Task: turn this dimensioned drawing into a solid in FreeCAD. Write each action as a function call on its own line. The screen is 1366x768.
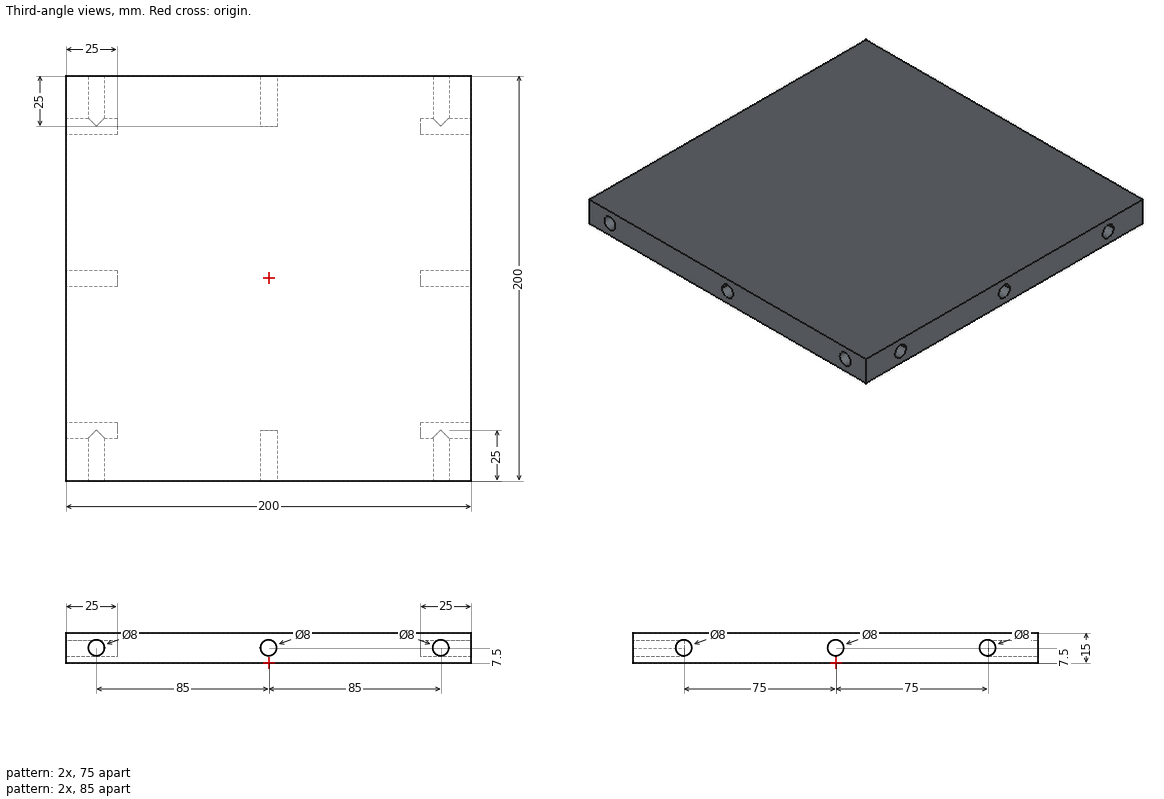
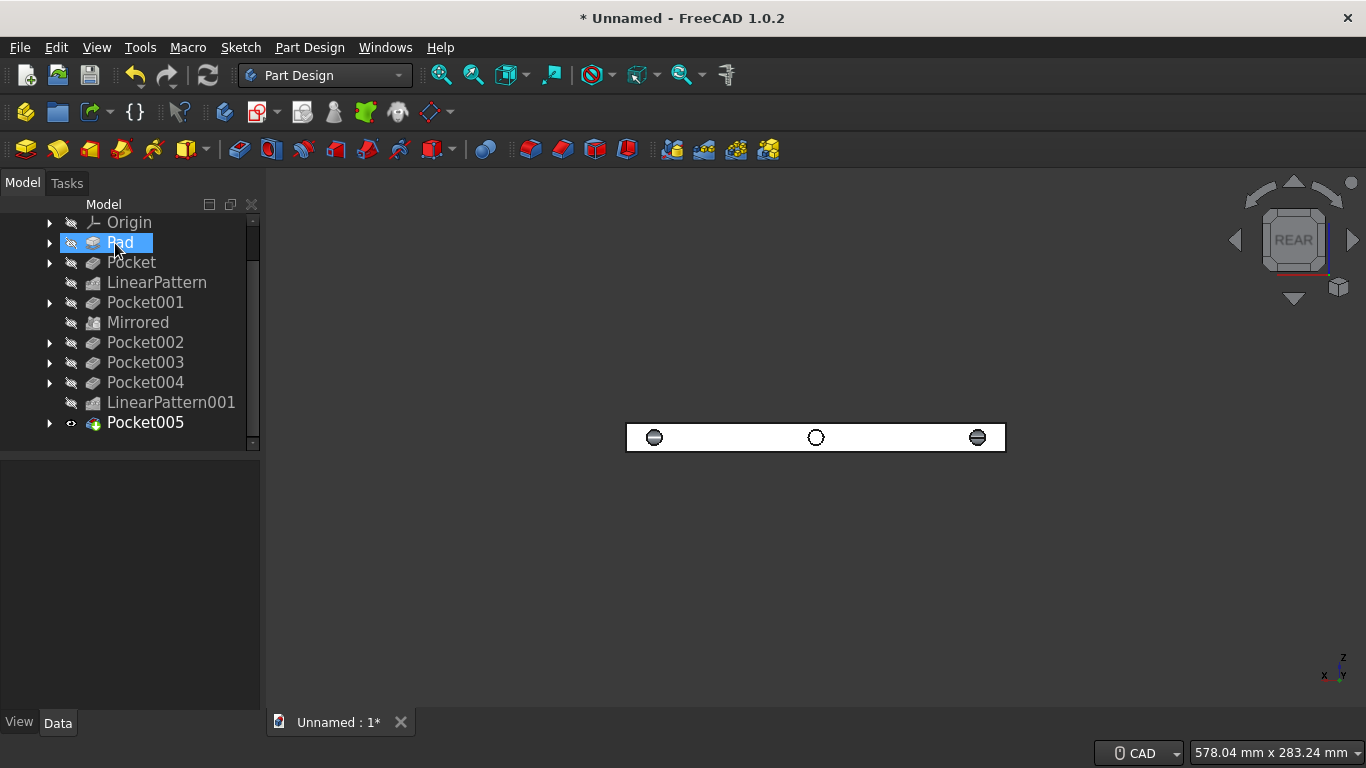
key(v)
key(f)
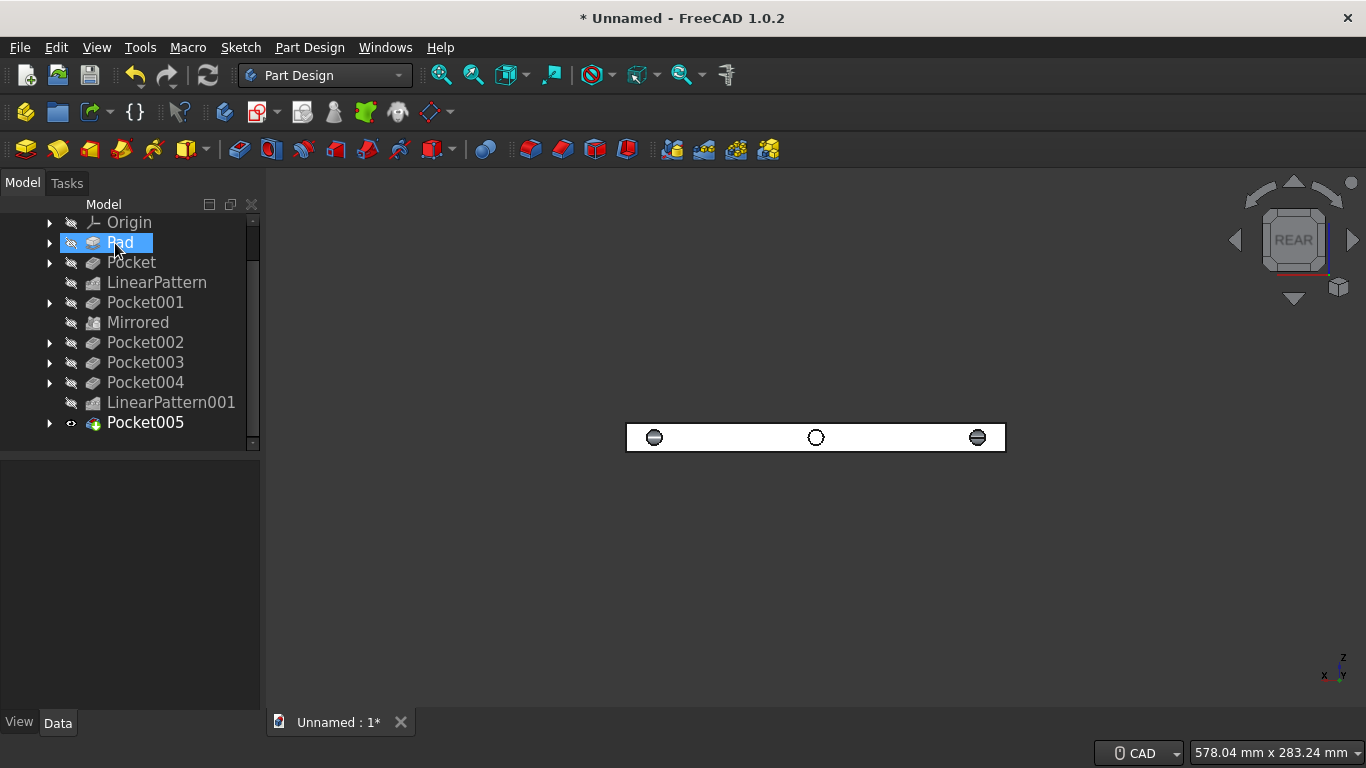
click(116, 383)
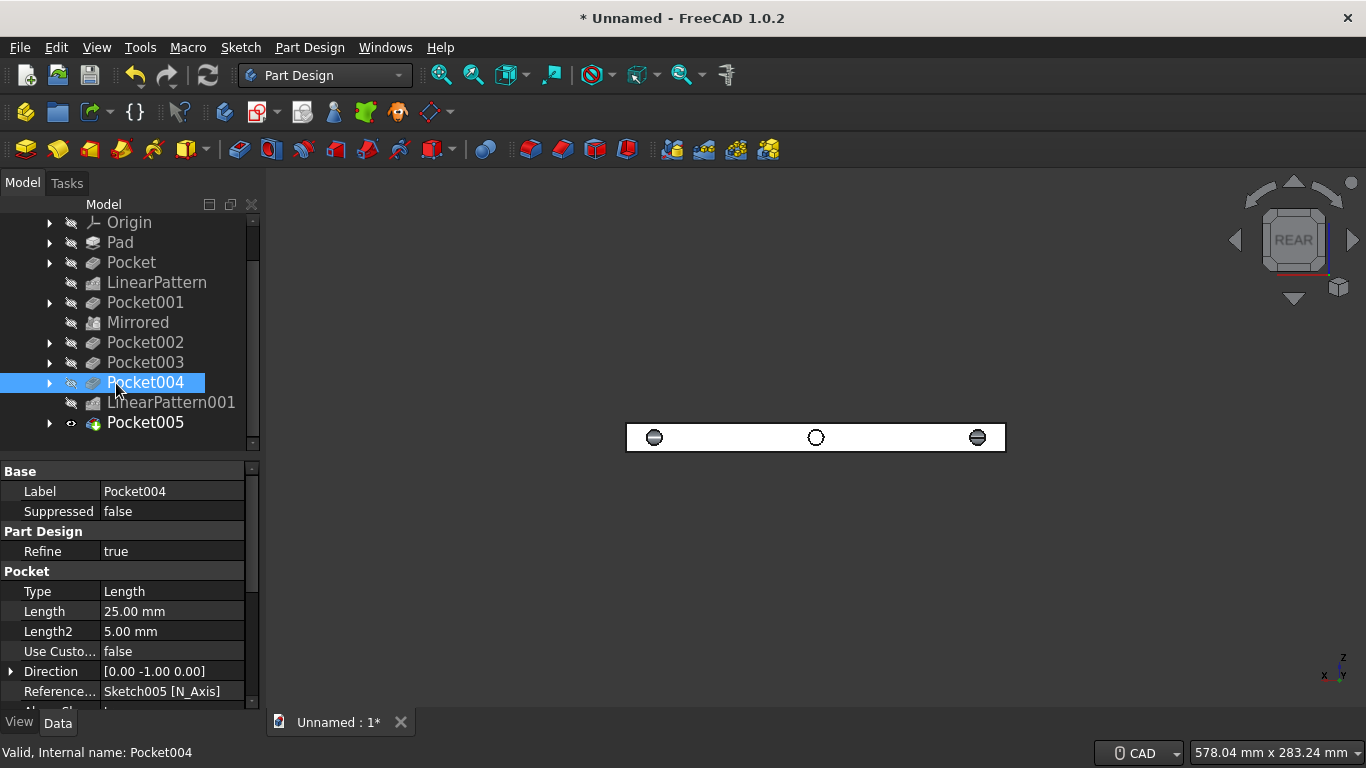
click(672, 150)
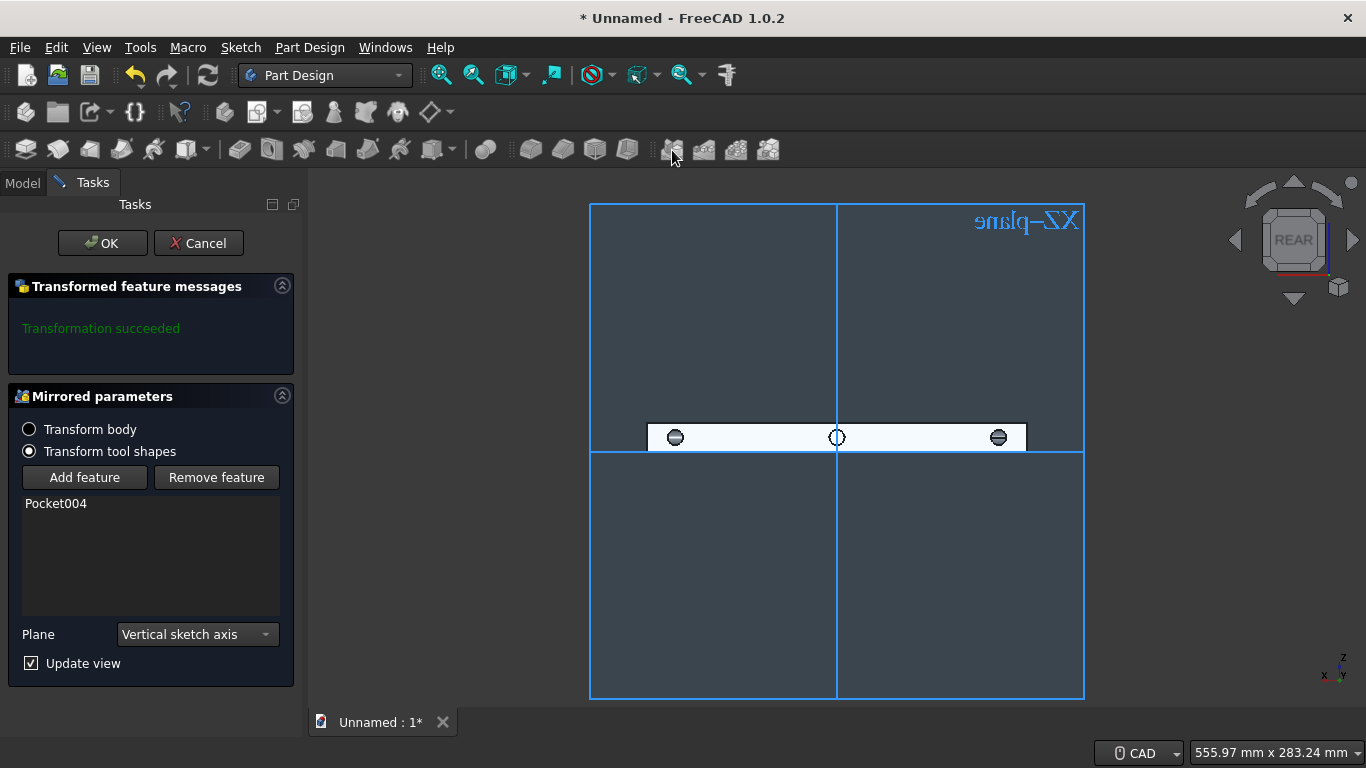
click(198, 634)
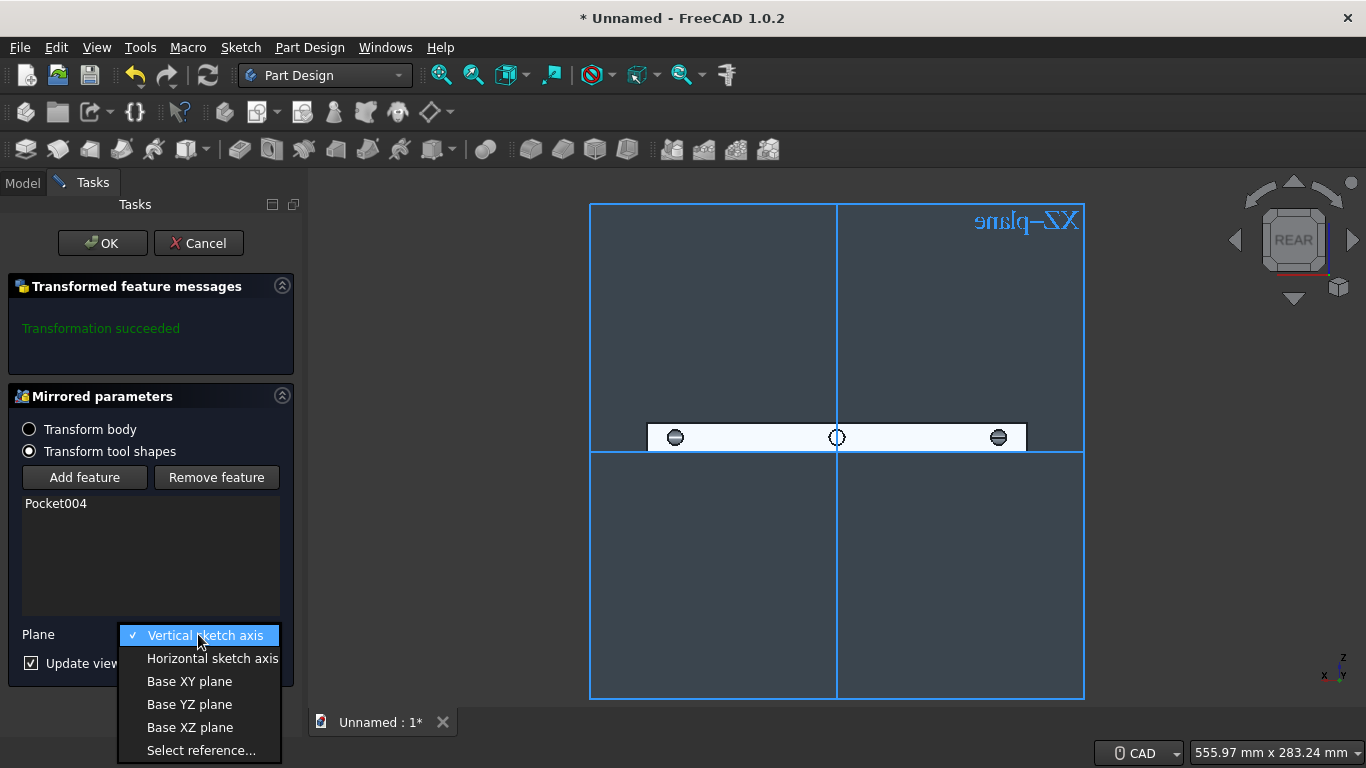
click(198, 728)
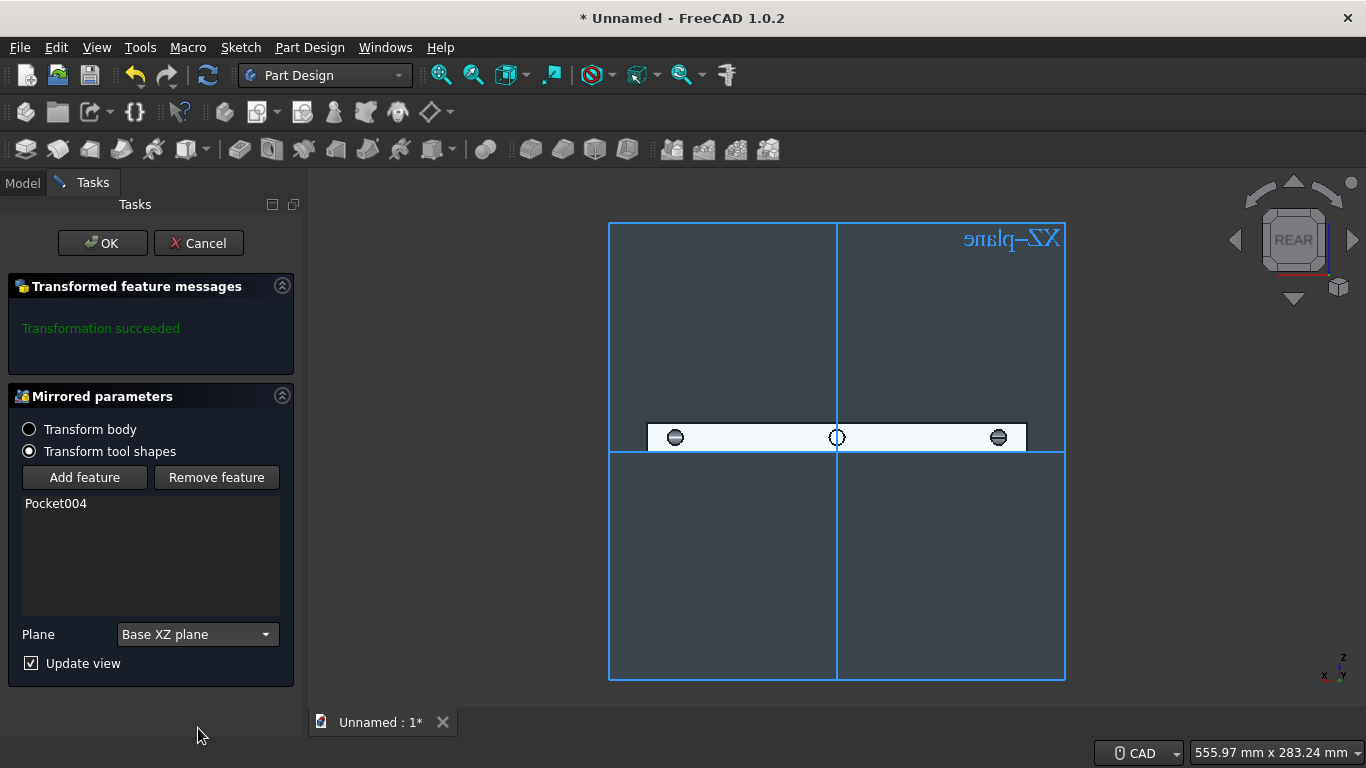
click(103, 243)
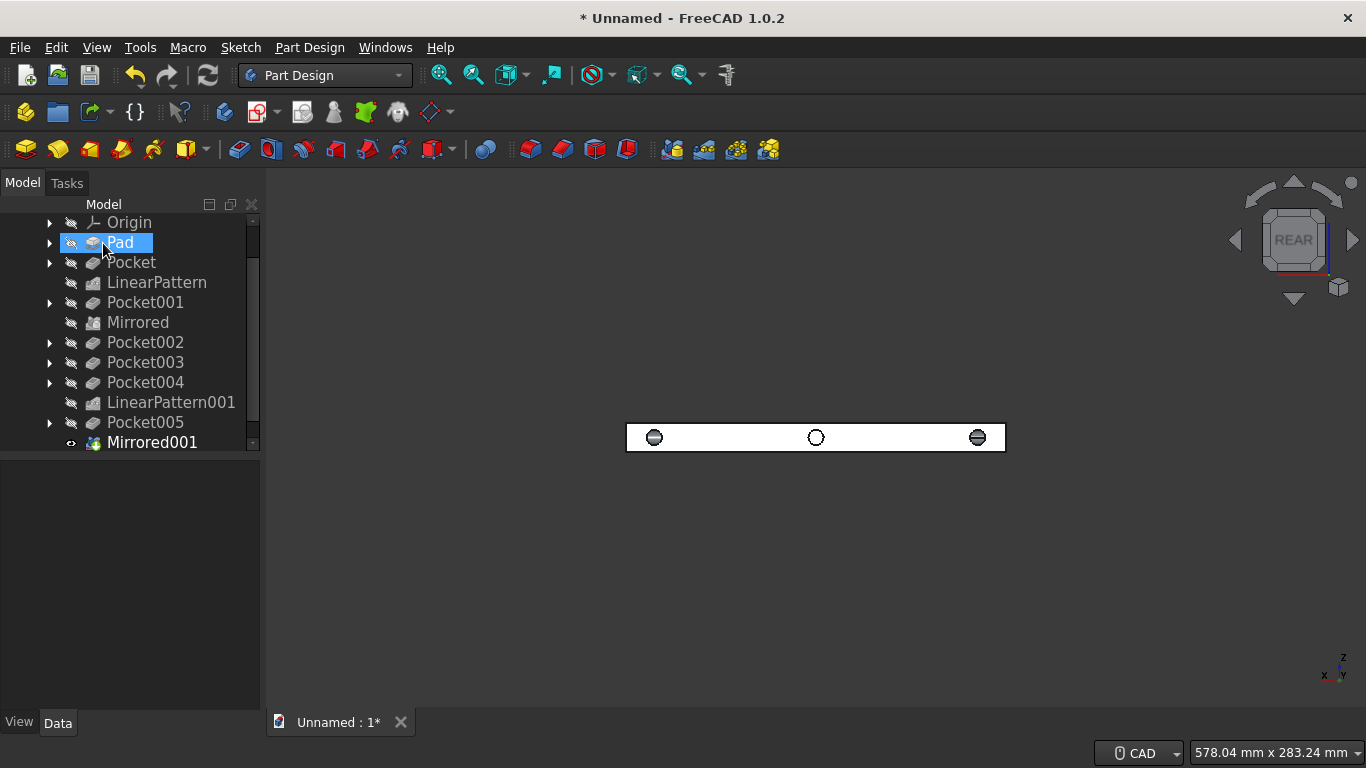
key(v)
key(f)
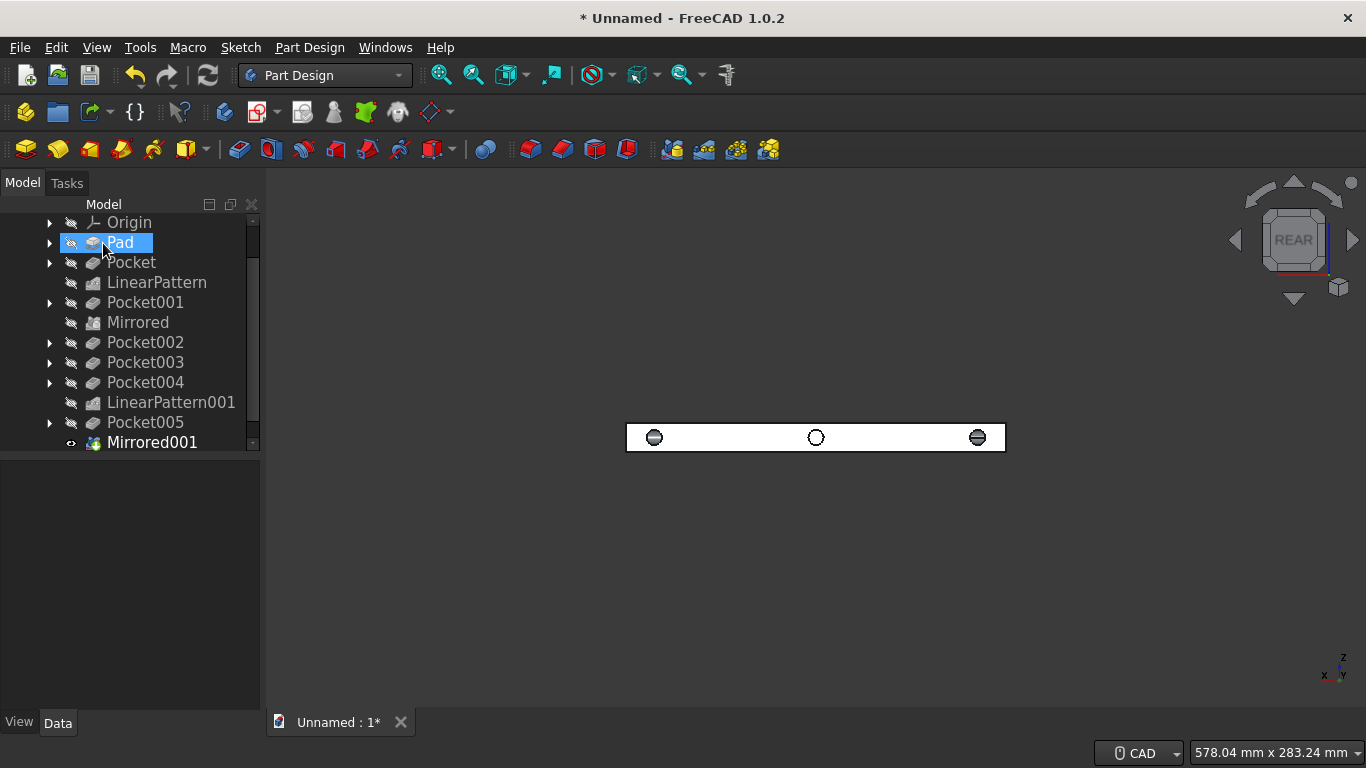
key(0)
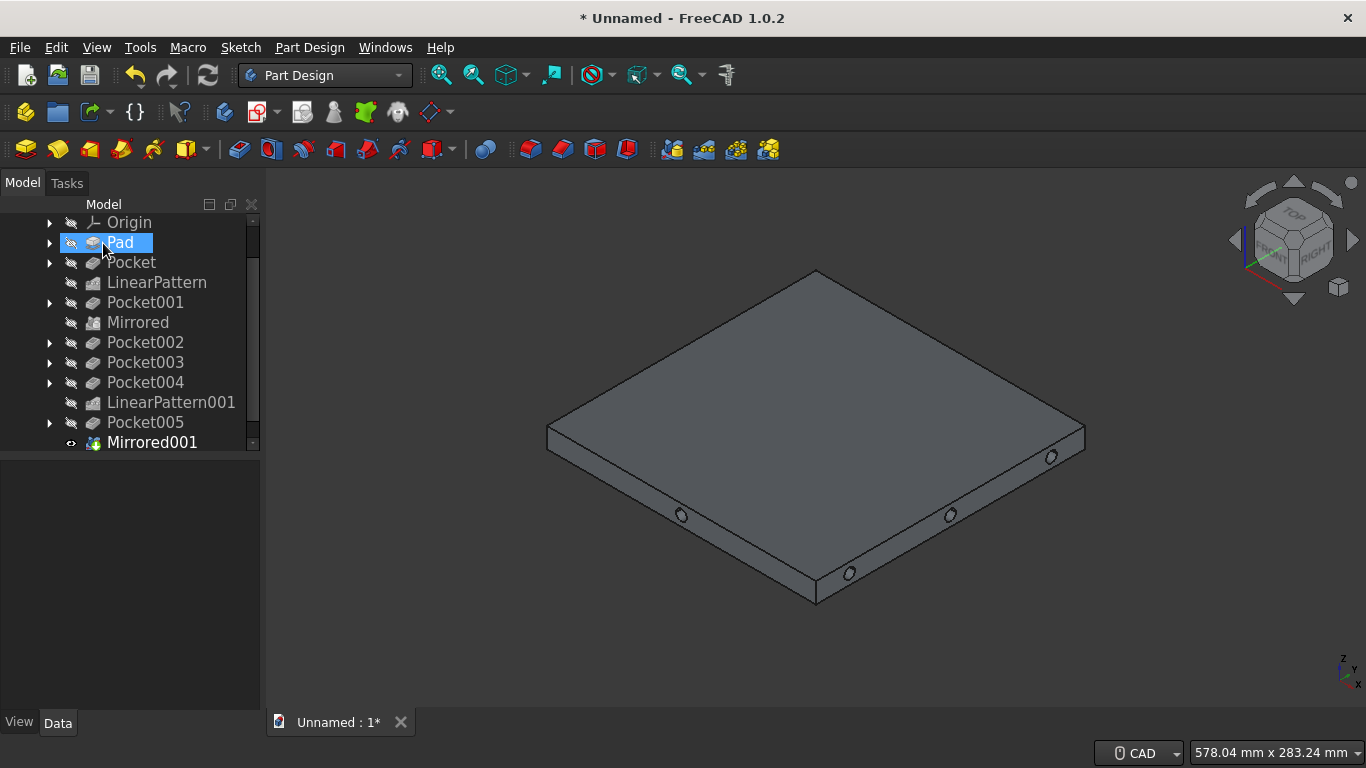
click(797, 581)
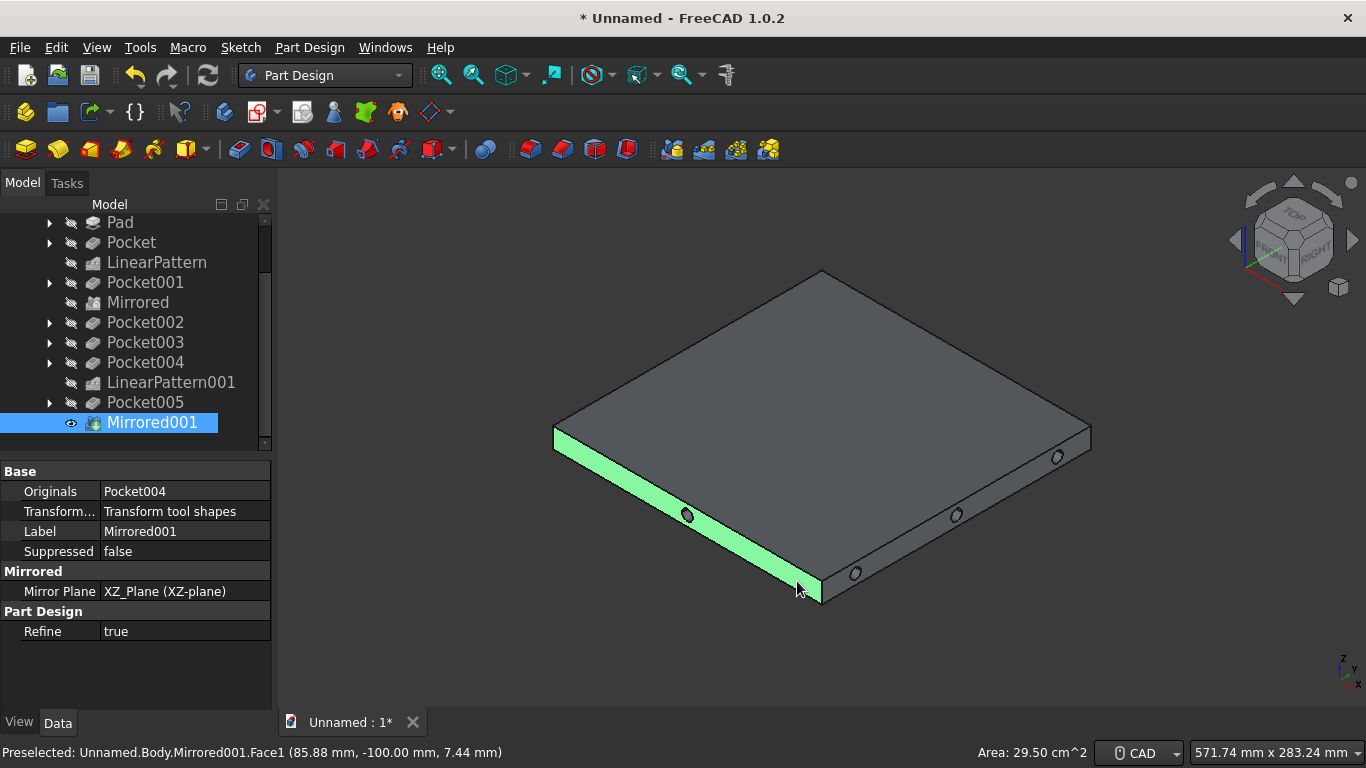
click(258, 112)